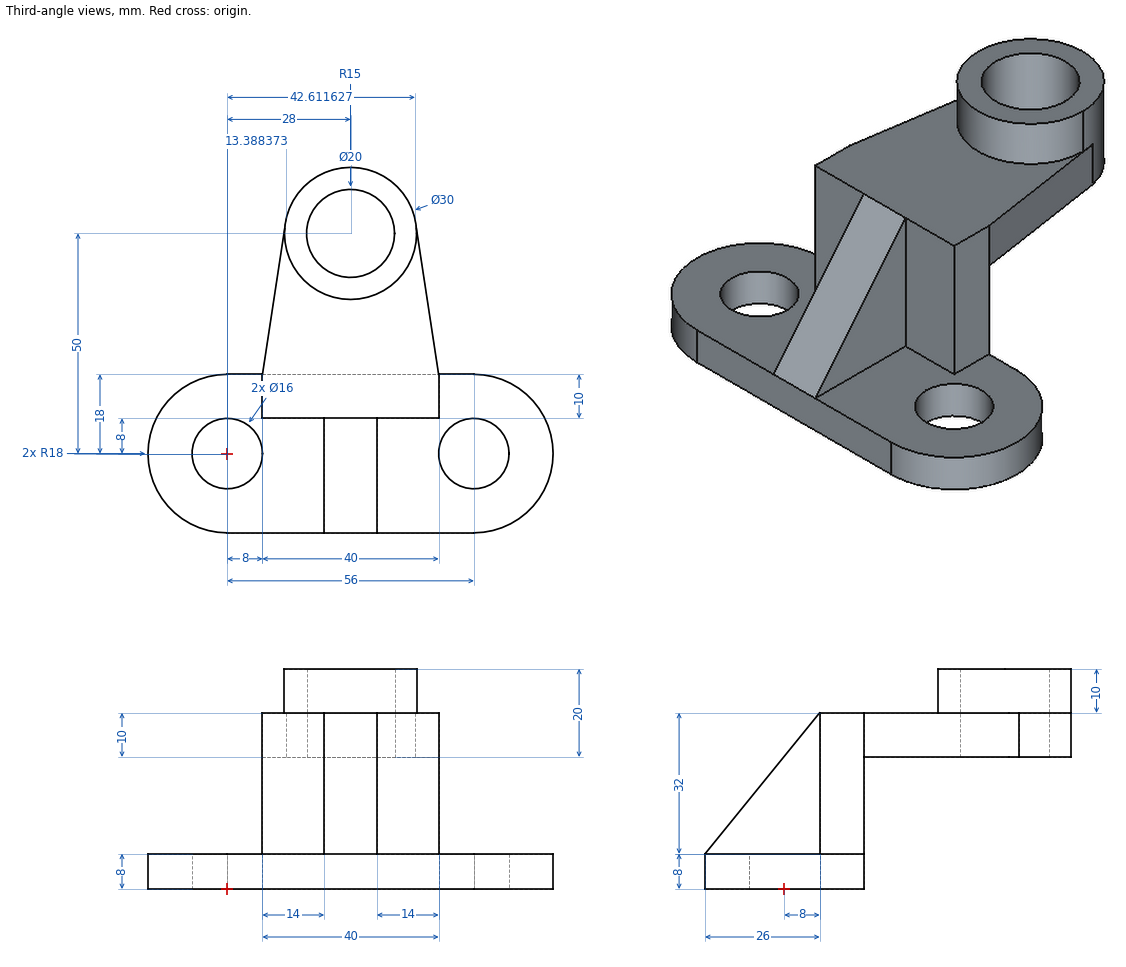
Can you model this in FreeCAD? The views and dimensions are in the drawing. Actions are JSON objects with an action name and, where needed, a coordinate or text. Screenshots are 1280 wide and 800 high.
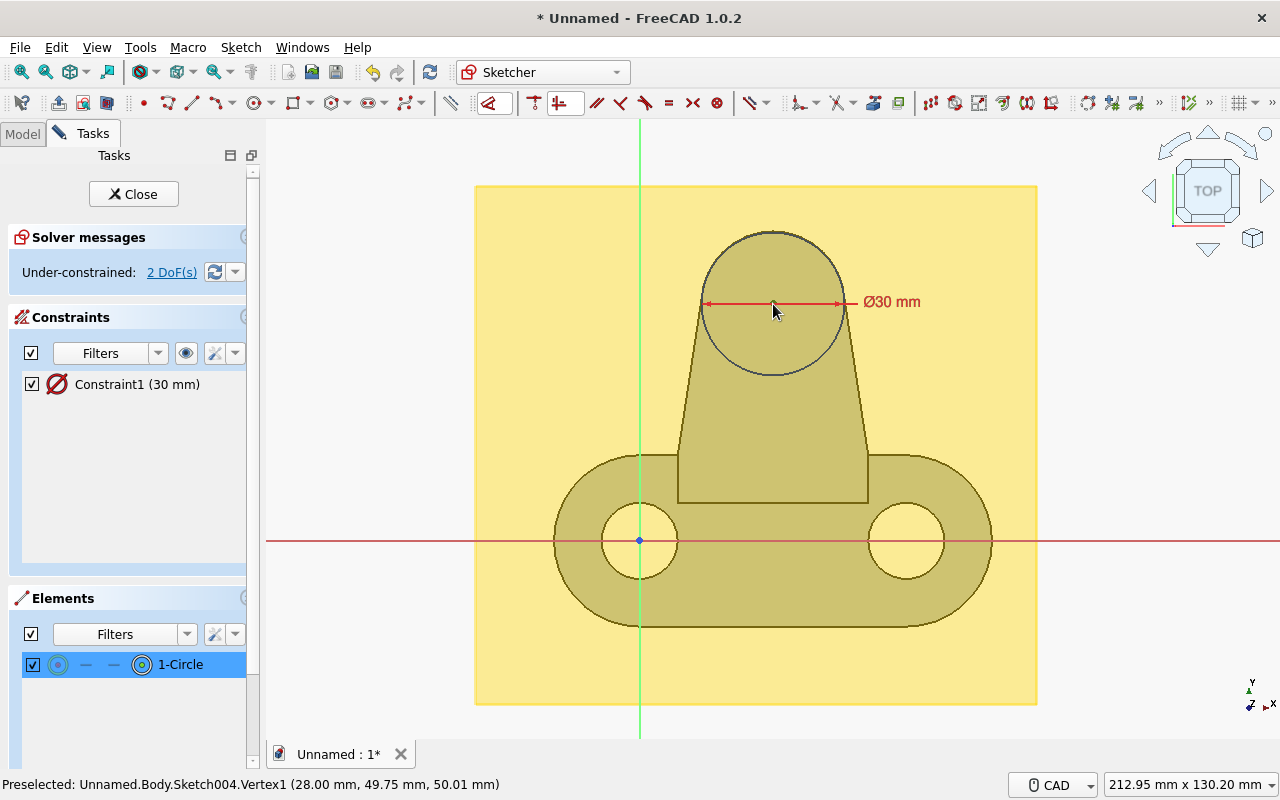
{"action": "left_click", "coordinate": [506, 104]}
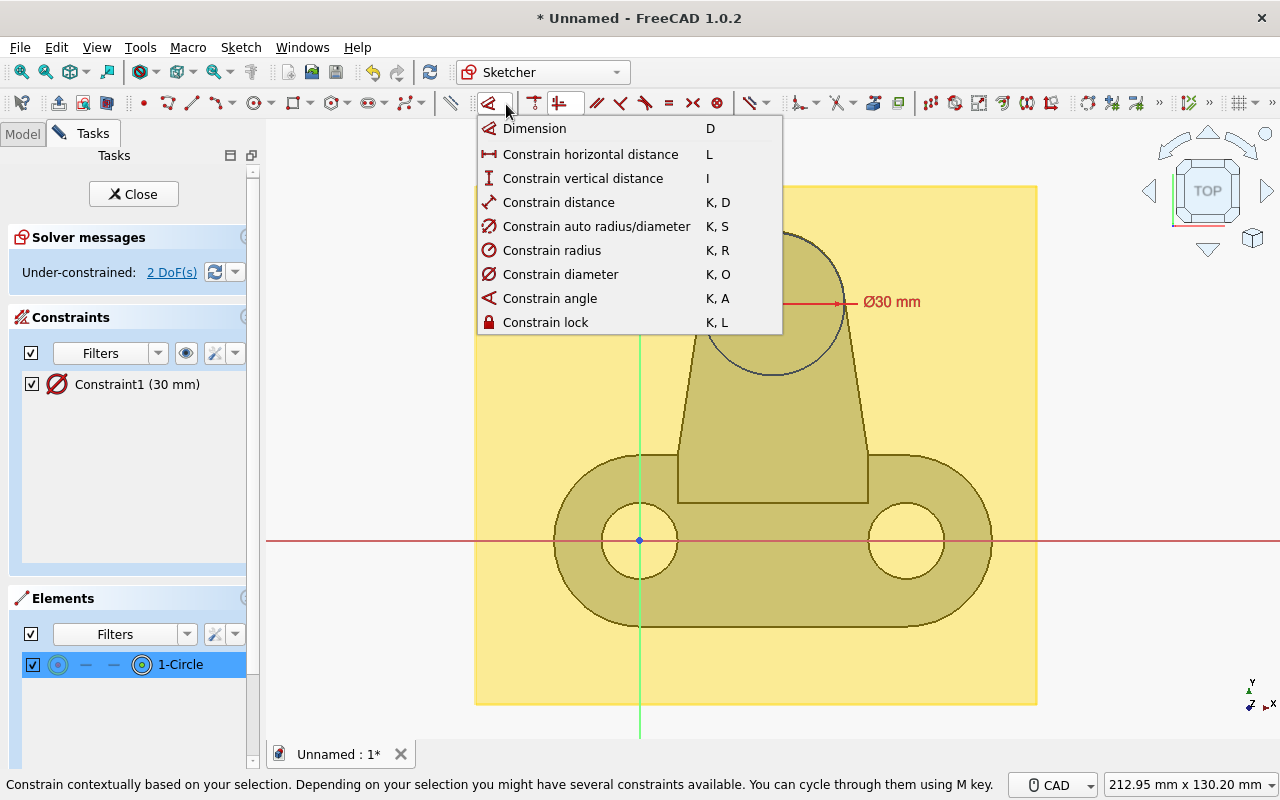
{"action": "left_click", "coordinate": [630, 154]}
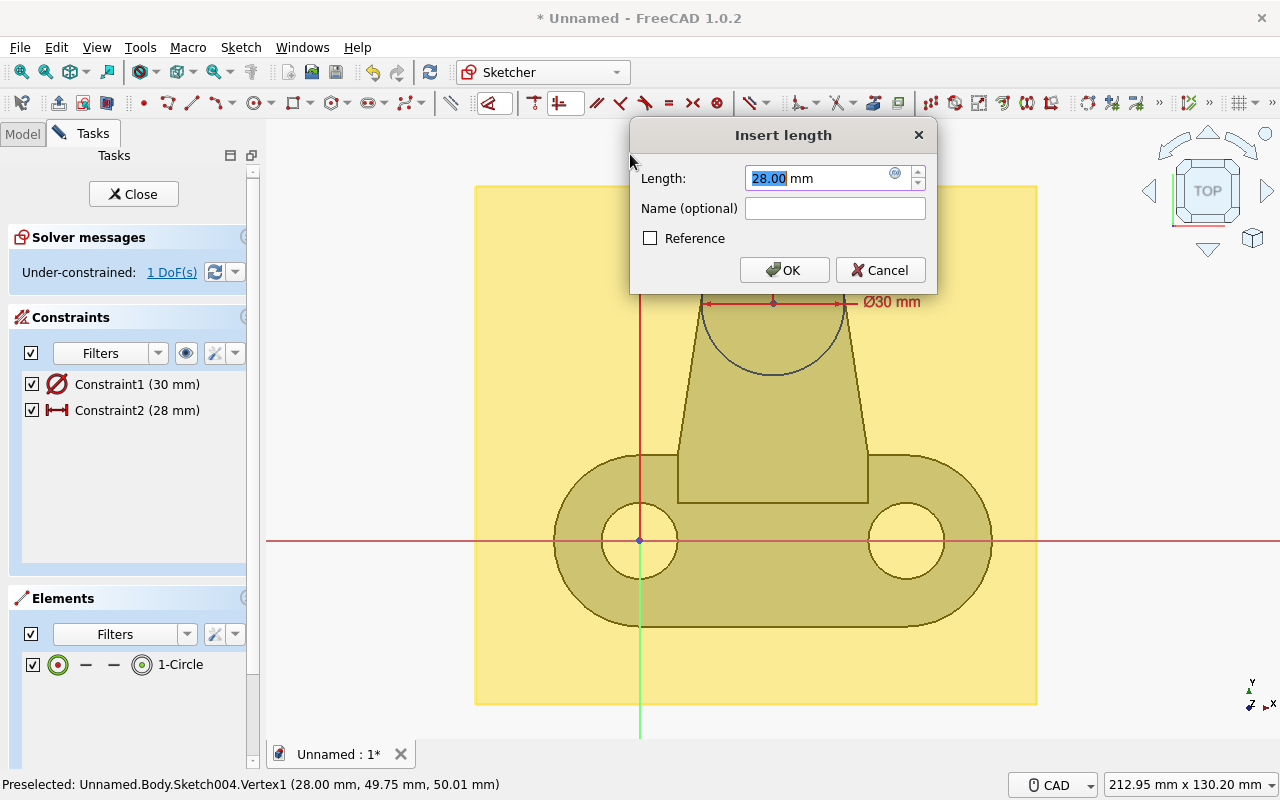
{"action": "type", "text": "28"}
{"action": "key", "text": "Return"}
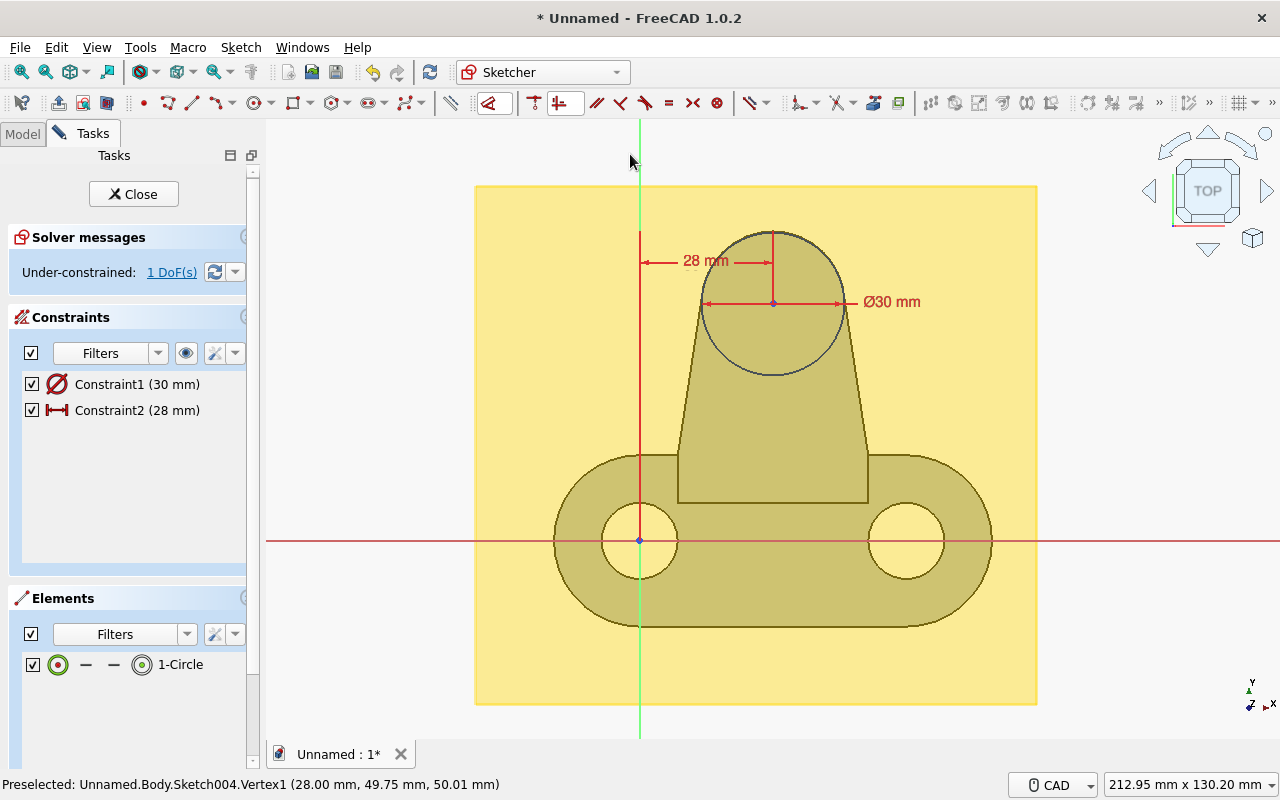
{"action": "left_click", "coordinate": [773, 304]}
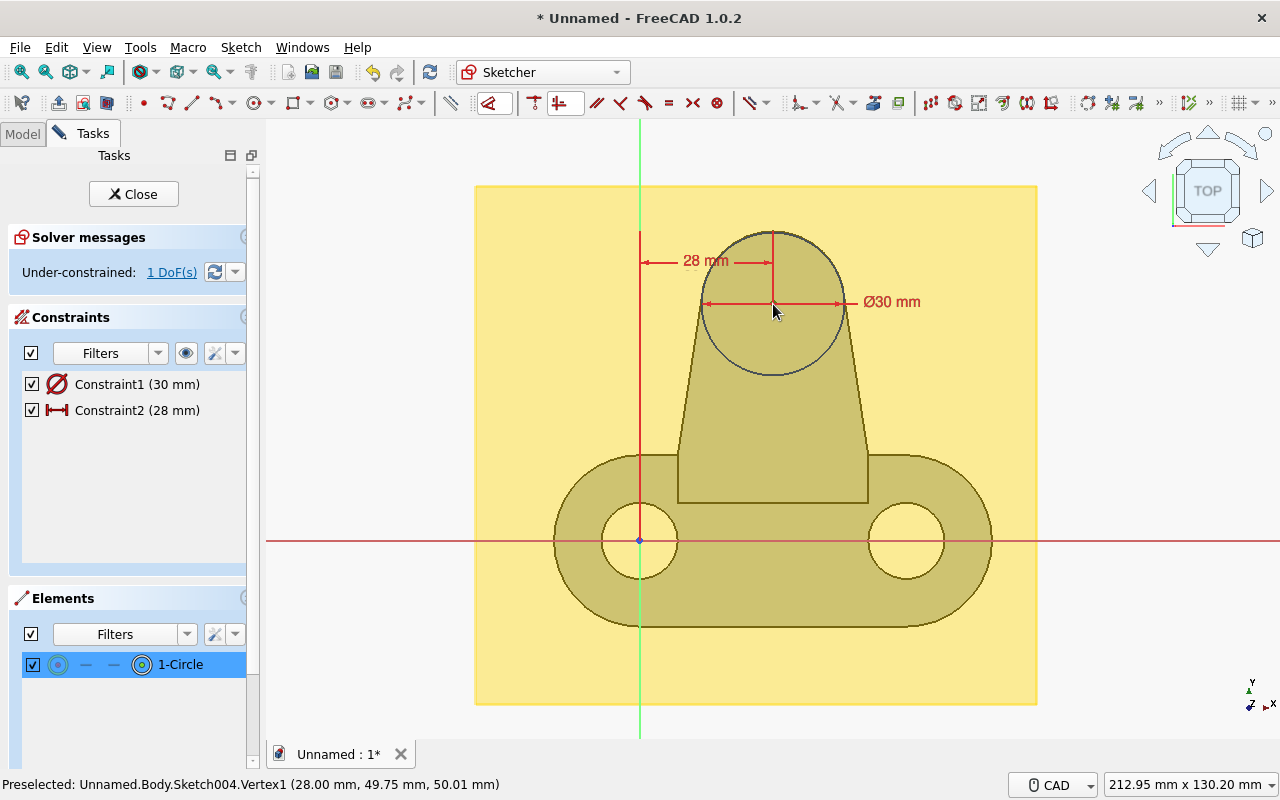
{"action": "key", "text": "i"}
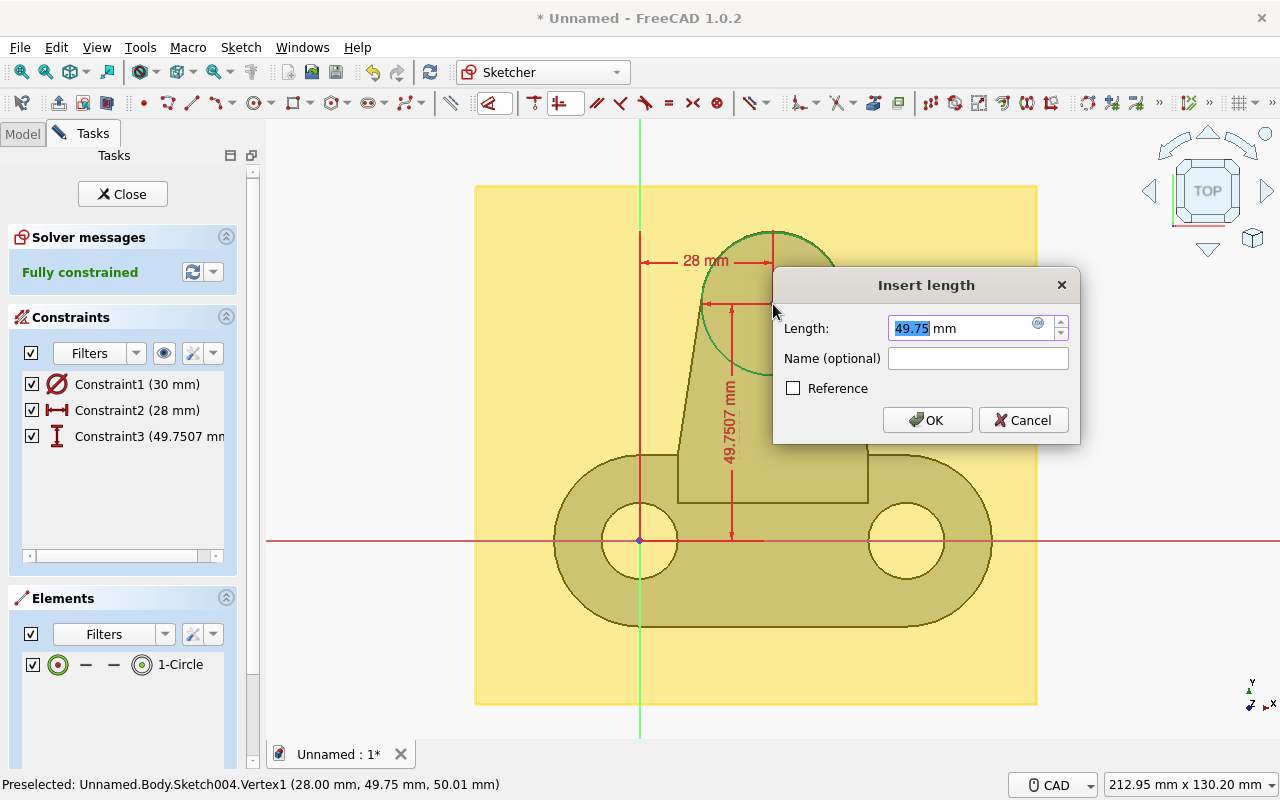
{"action": "type", "text": "50"}
{"action": "key", "text": "Return"}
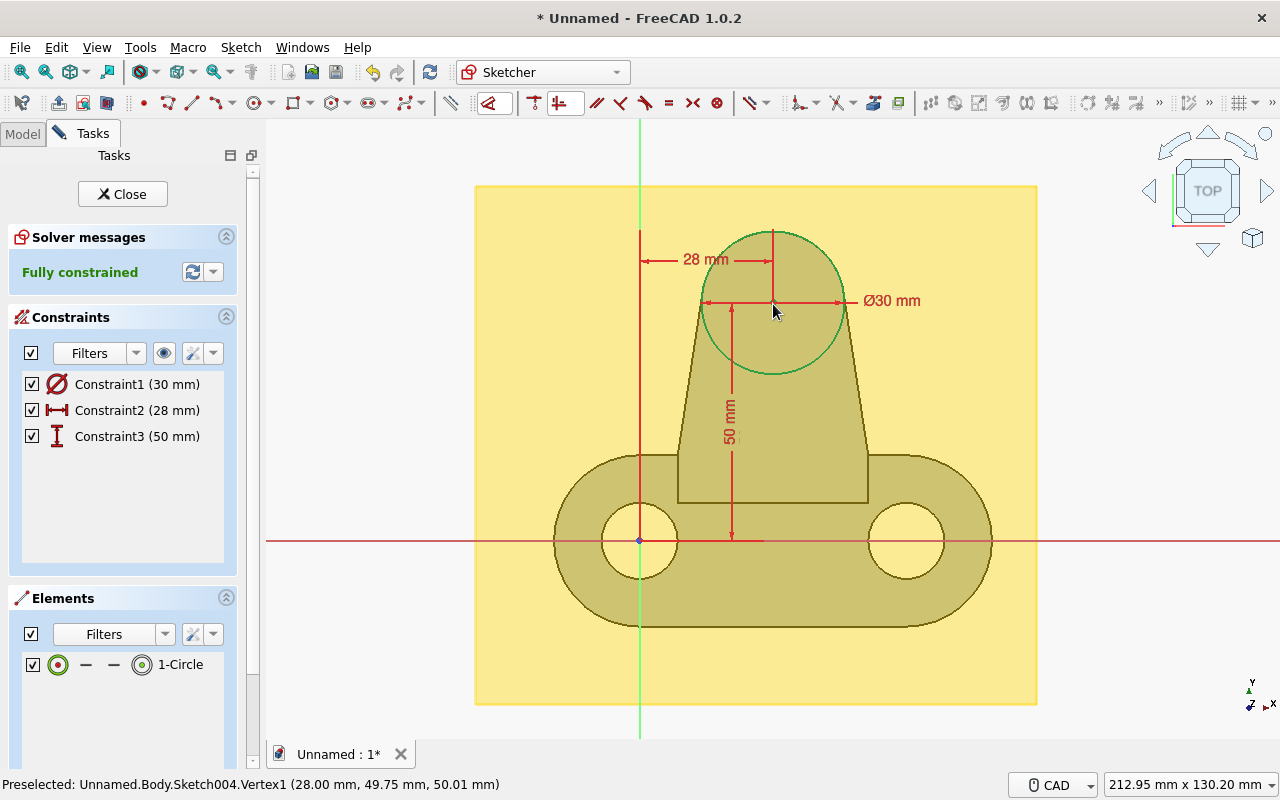
{"action": "left_click", "coordinate": [123, 194]}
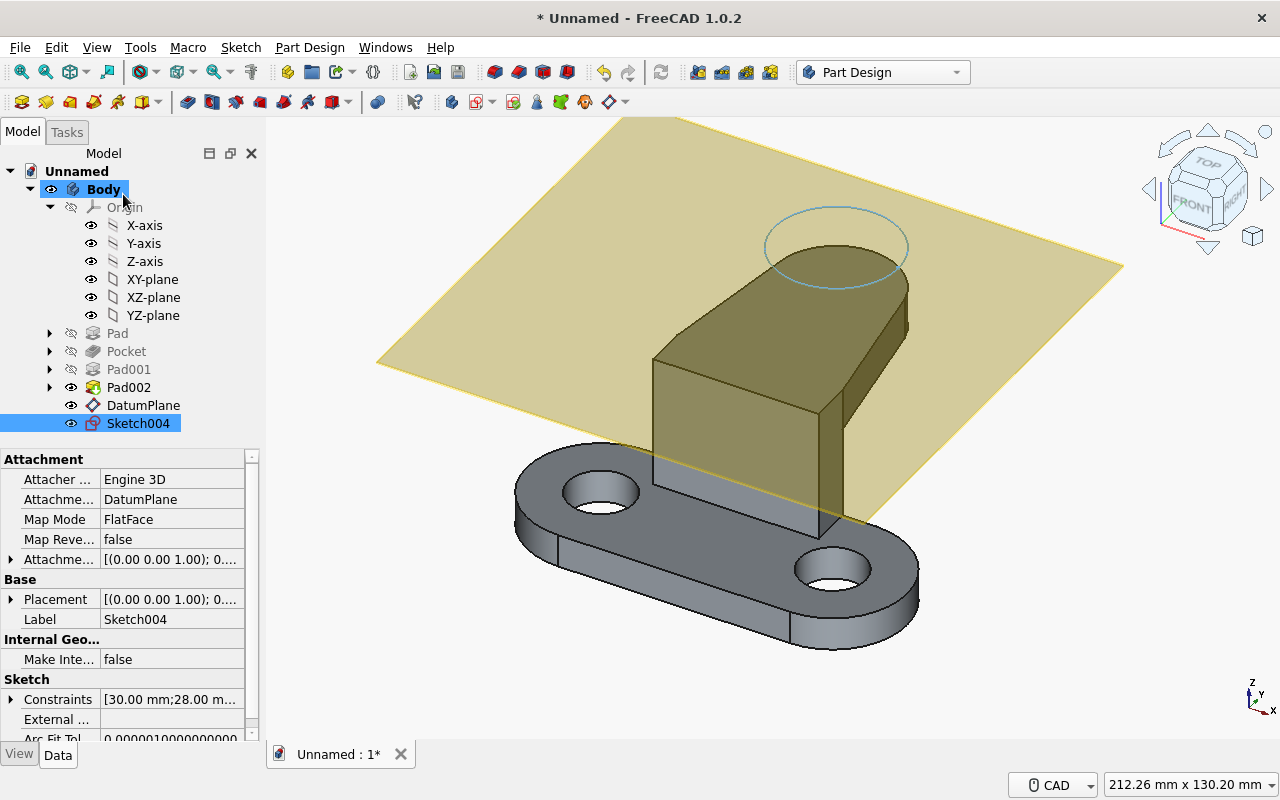
{"action": "left_click", "coordinate": [22, 102]}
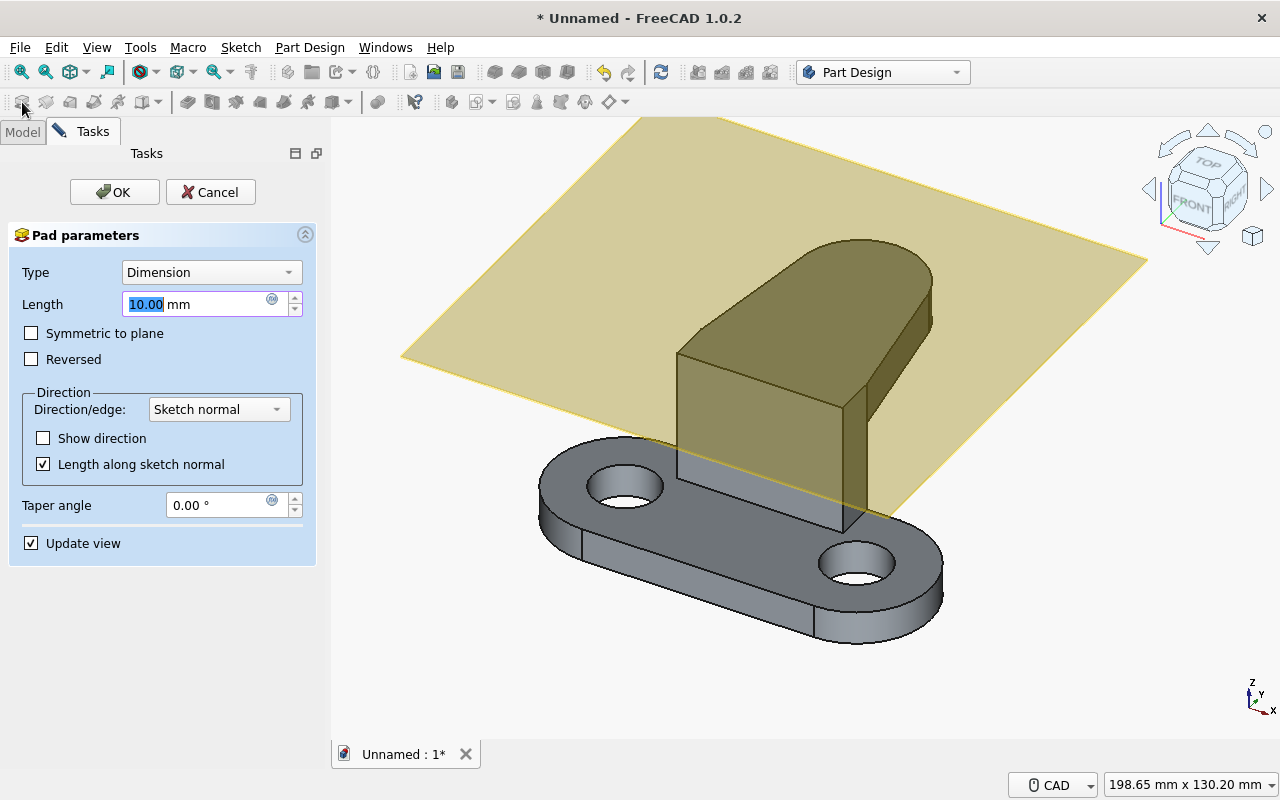
{"action": "type", "text": "10"}
{"action": "key", "text": "Tab"}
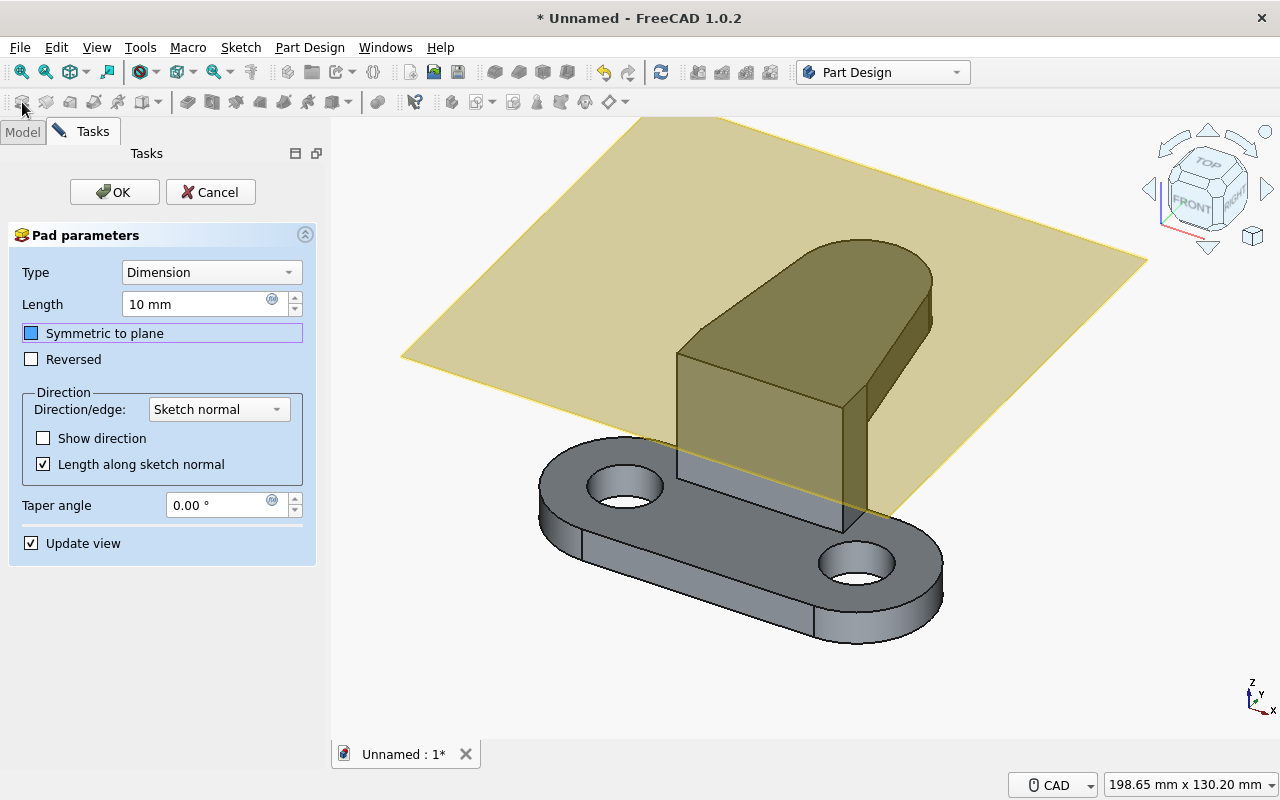
{"action": "left_click", "coordinate": [30, 359]}